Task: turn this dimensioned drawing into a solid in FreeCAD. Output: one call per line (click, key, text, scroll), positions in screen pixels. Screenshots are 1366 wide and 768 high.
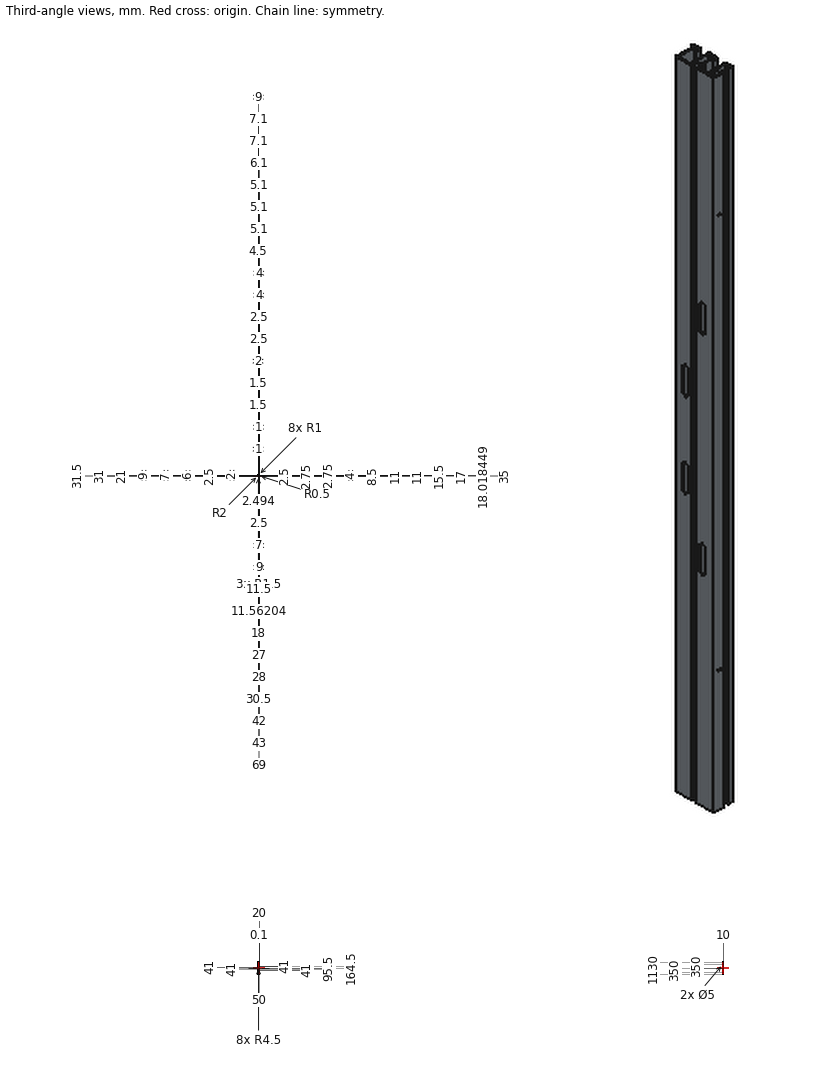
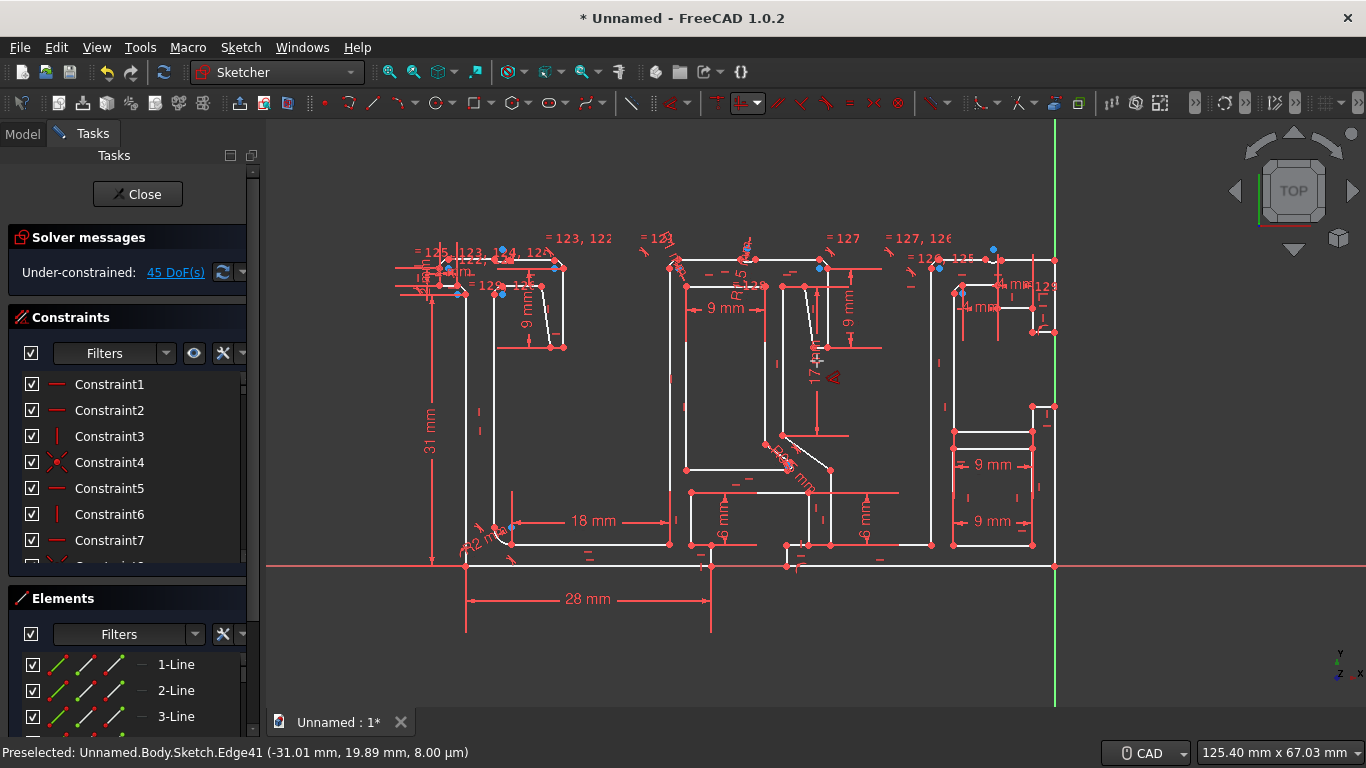
click(953, 478)
click(987, 497)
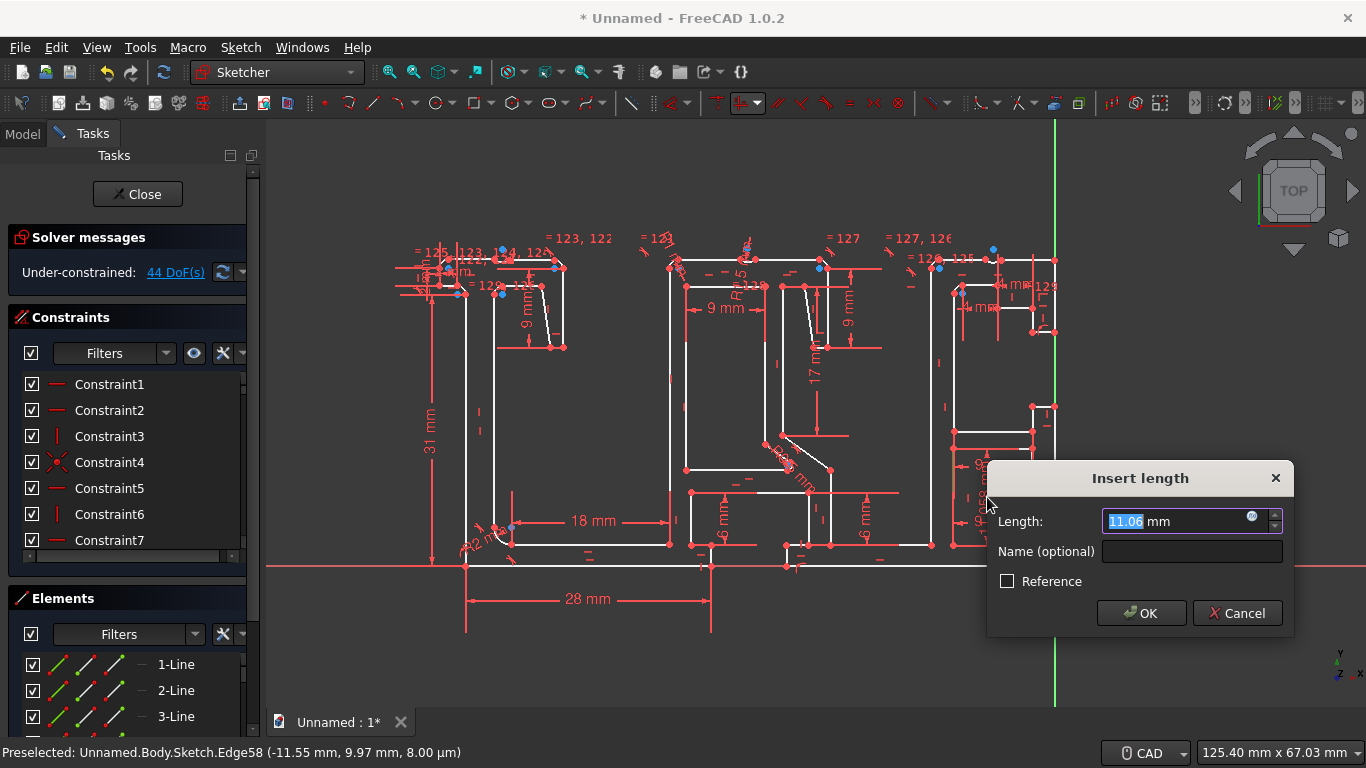
text(11)
key(Return)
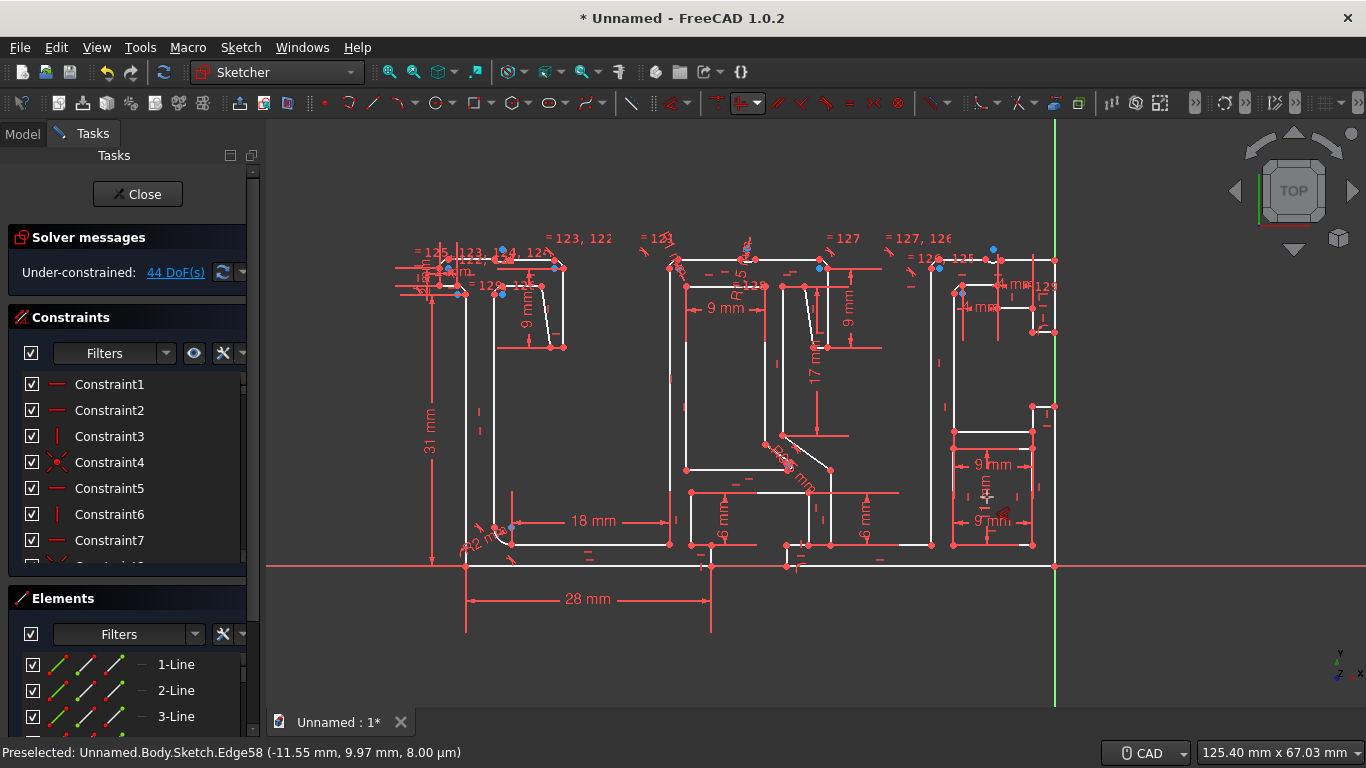
click(686, 415)
click(652, 378)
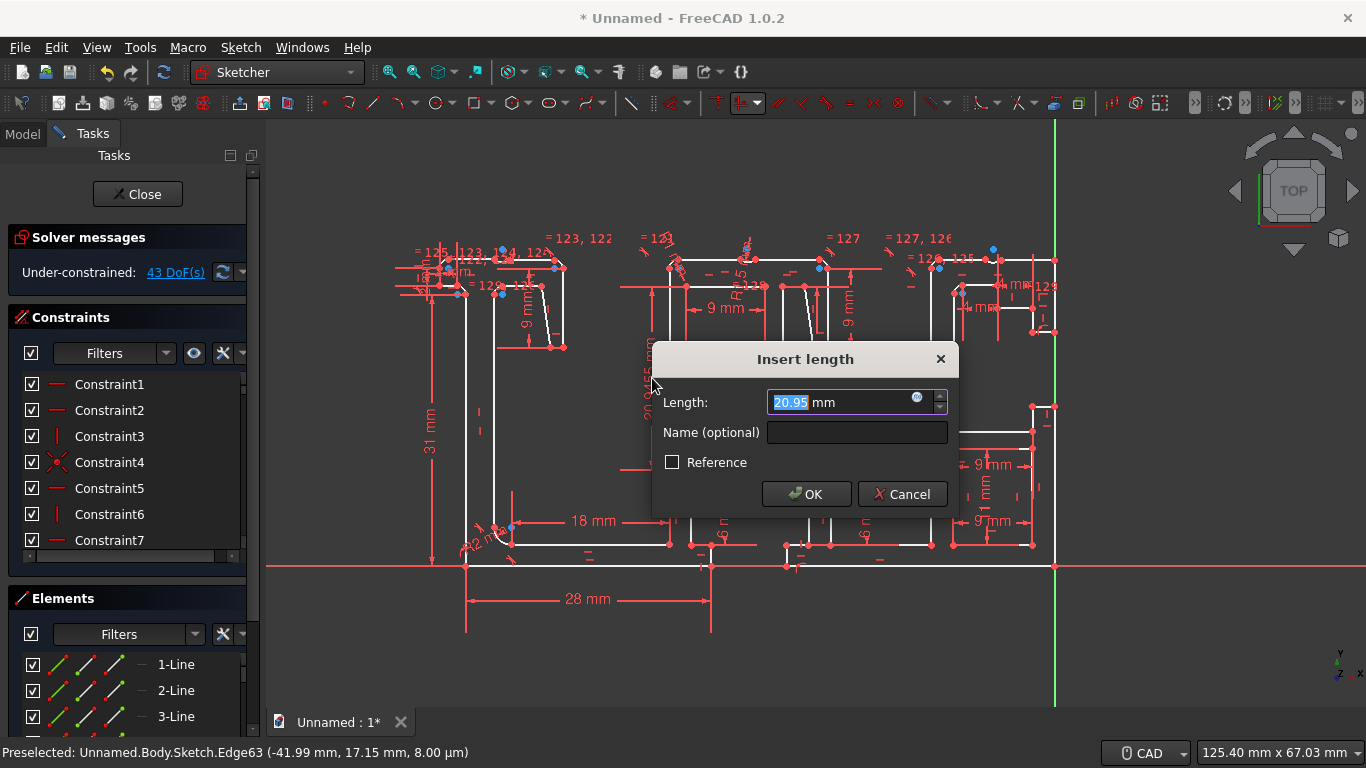
text(21)
key(Return)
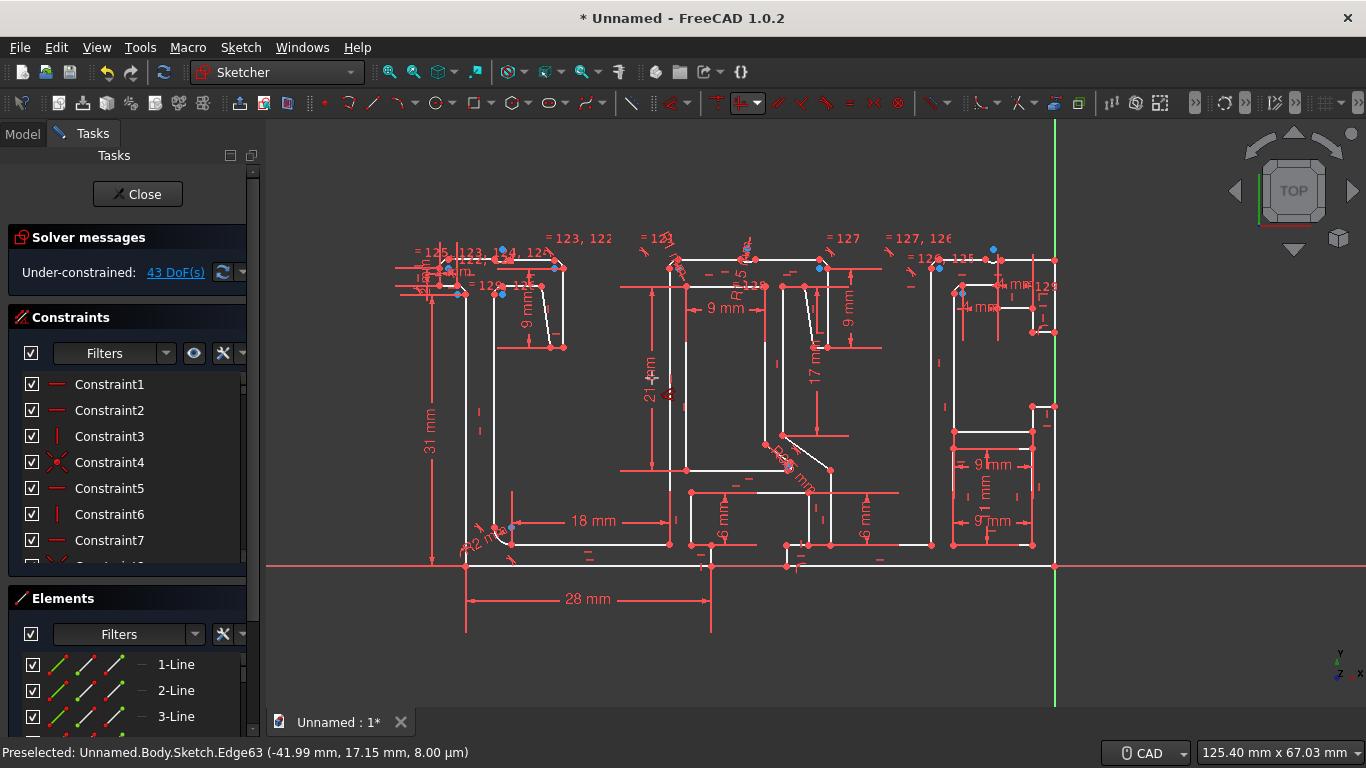
scroll(544, 305, up, 8)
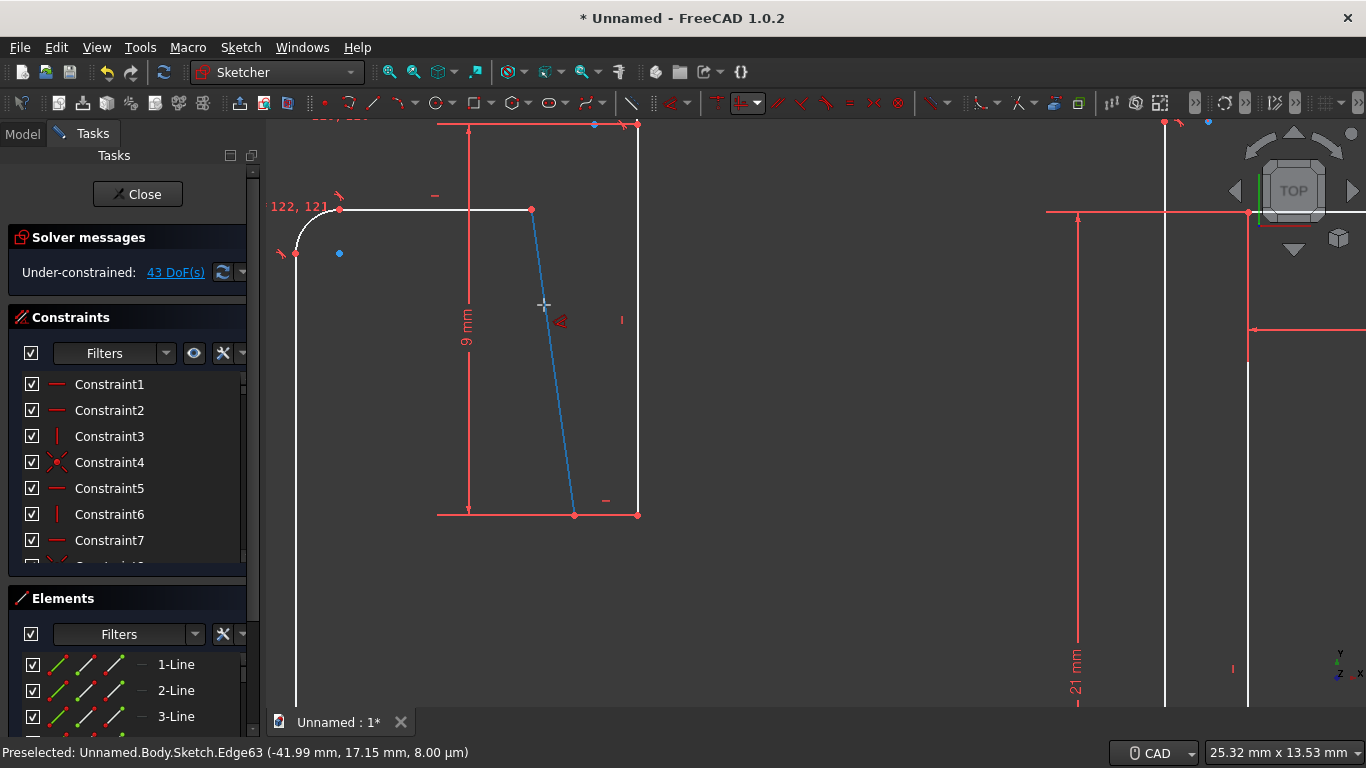
click(545, 302)
click(553, 176)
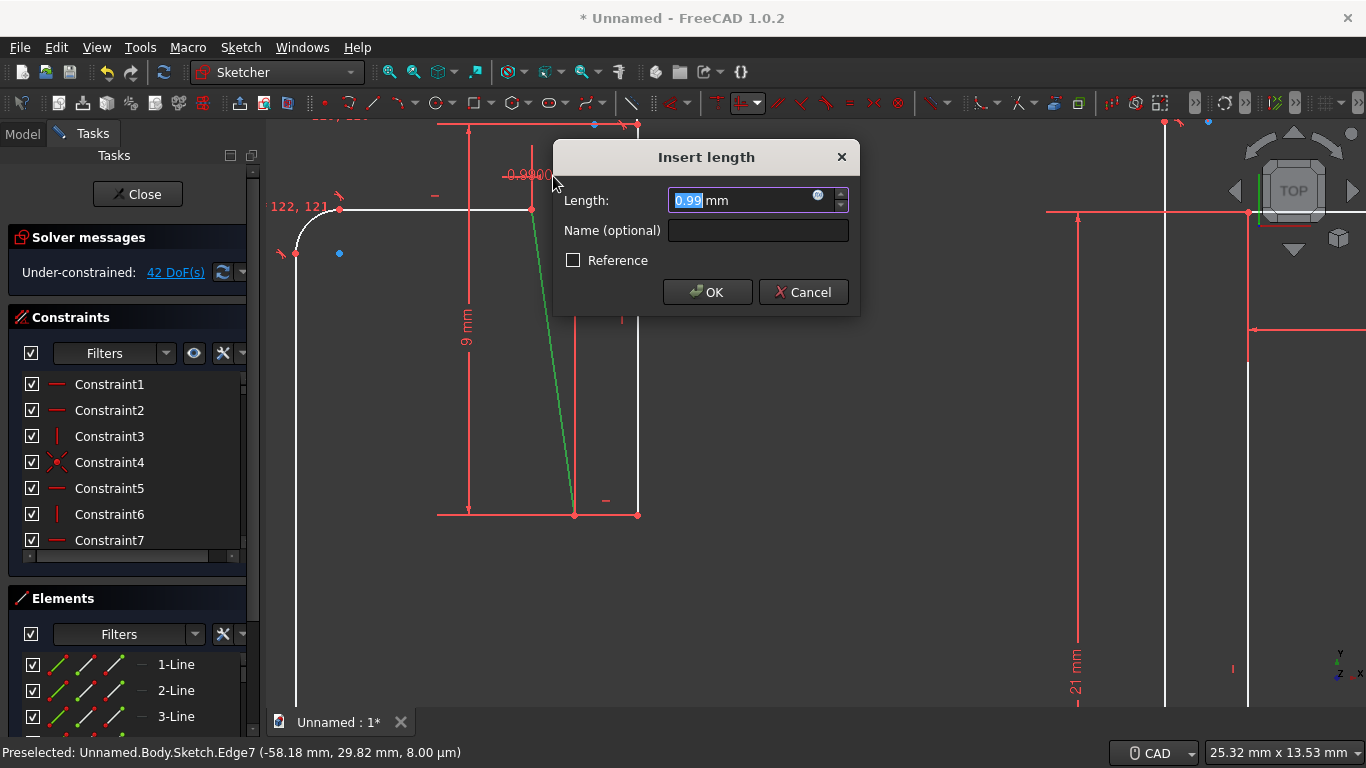
text(1)
key(Return)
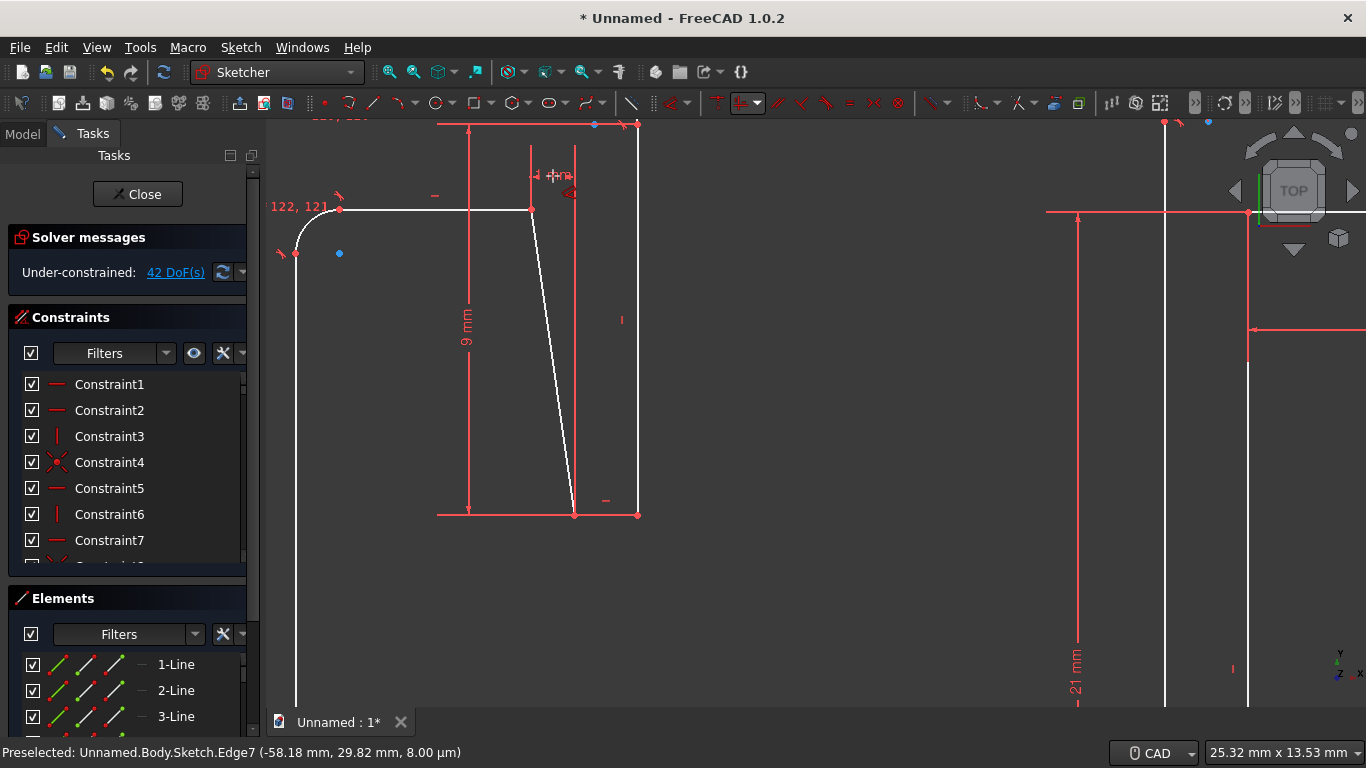
scroll(544, 305, down, 8)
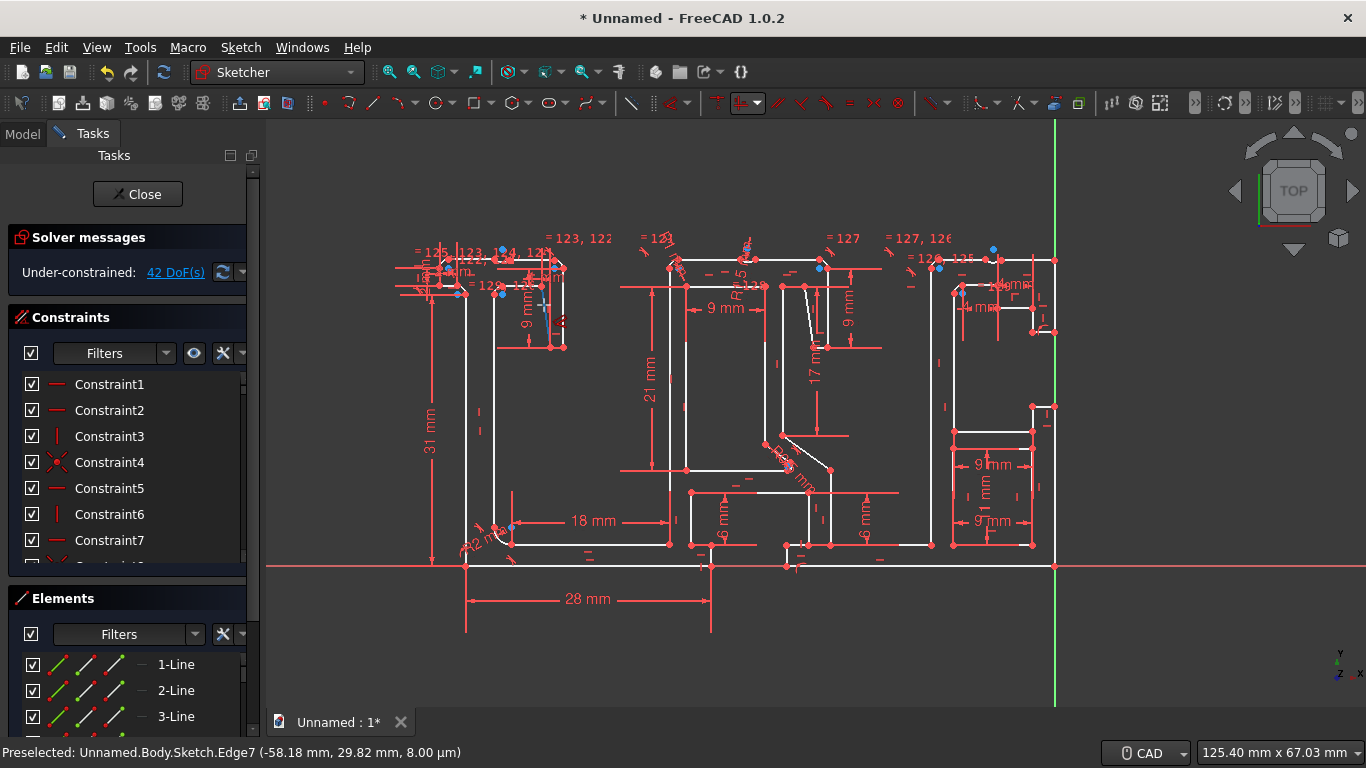
click(544, 305)
click(508, 331)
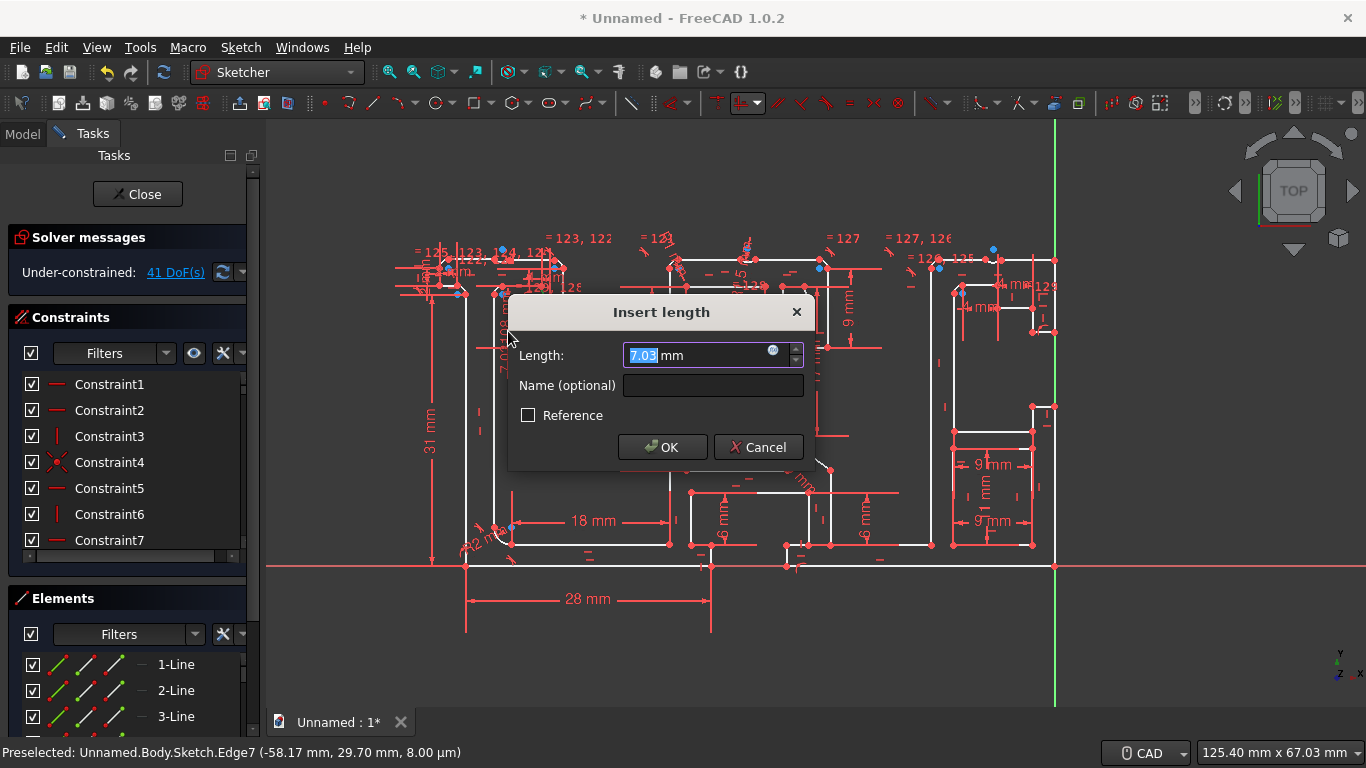
text(7)
key(Return)